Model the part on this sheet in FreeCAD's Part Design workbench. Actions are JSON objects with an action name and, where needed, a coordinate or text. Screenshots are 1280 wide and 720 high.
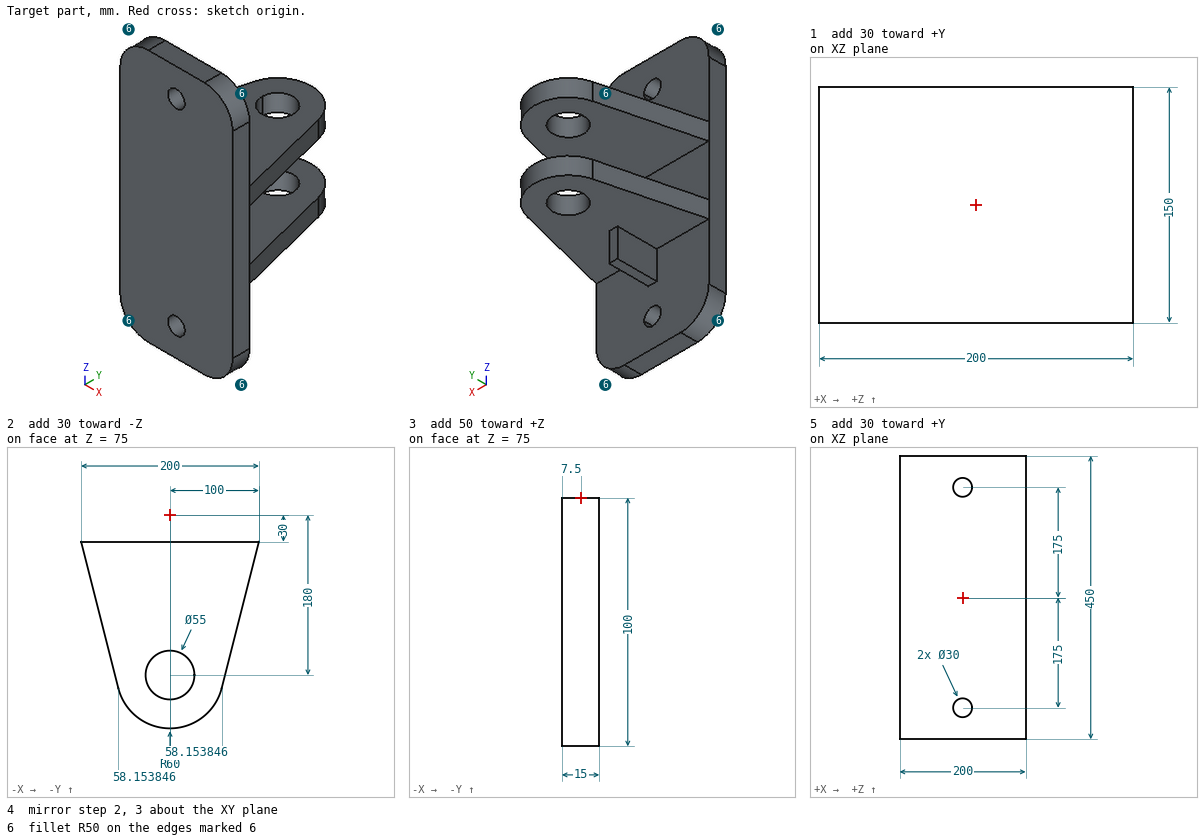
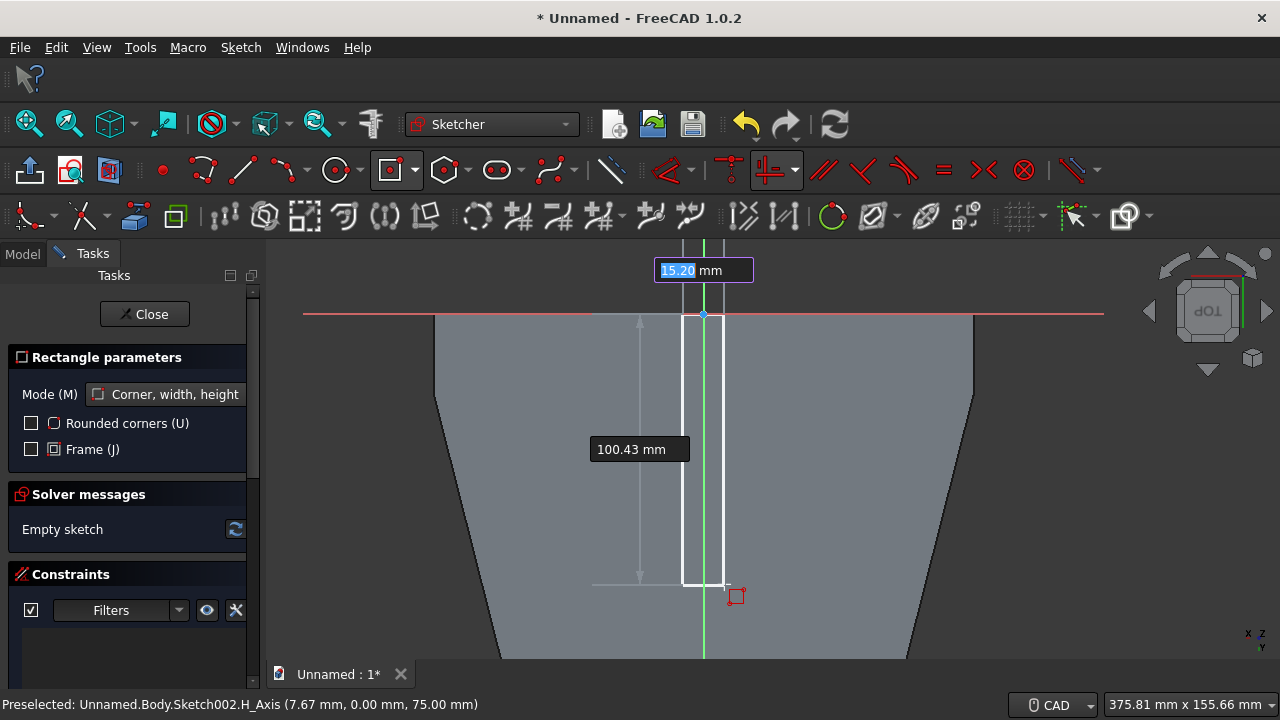
{"action": "type", "text": "15"}
{"action": "key", "text": "Tab"}
{"action": "type", "text": "100"}
{"action": "key", "text": "Return"}
{"action": "key", "text": "Escape"}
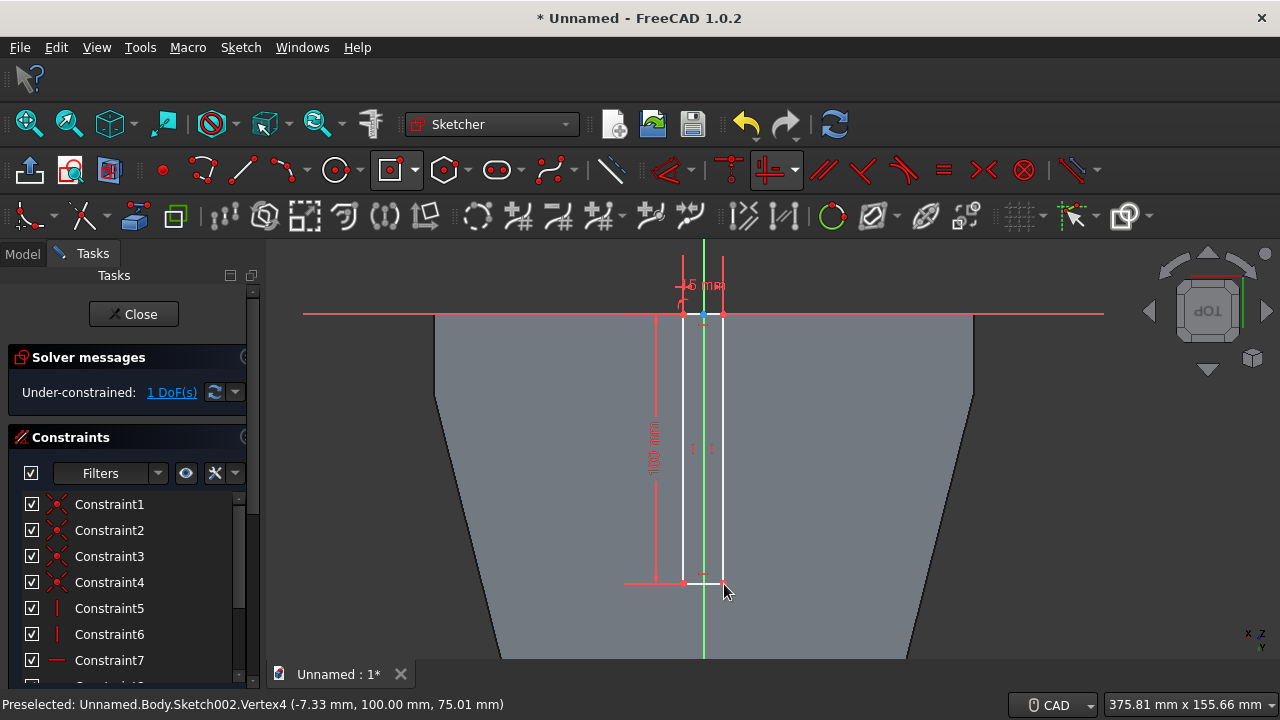
{"action": "key", "text": "d"}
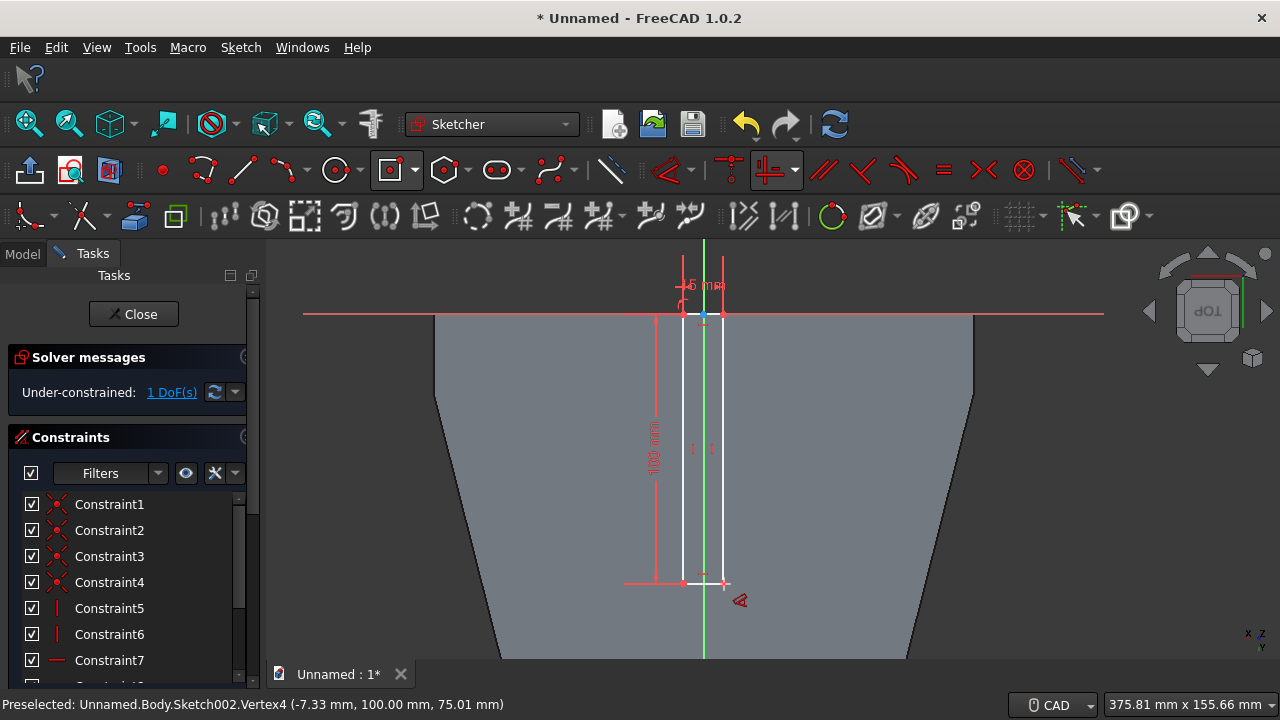
{"action": "scroll", "coordinate": [683, 314], "scroll_direction": "up", "scroll_amount": 4}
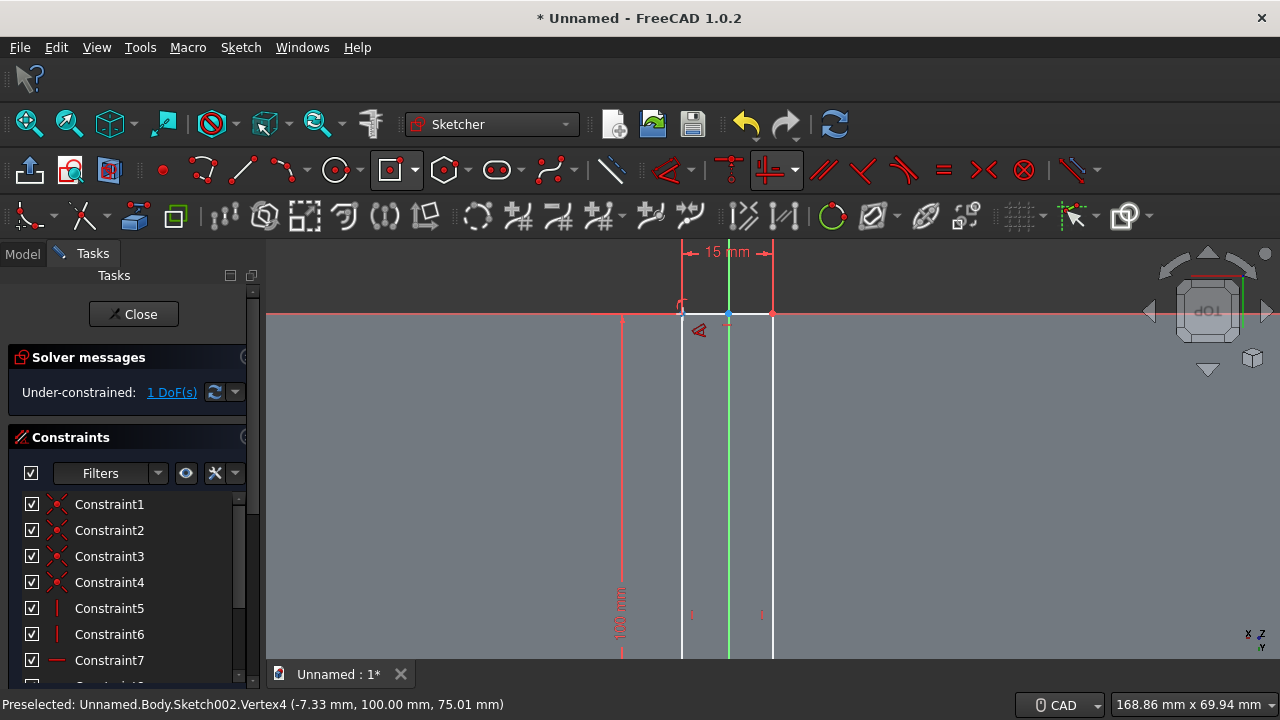
{"action": "left_click", "coordinate": [682, 314]}
{"action": "left_click", "coordinate": [706, 280]}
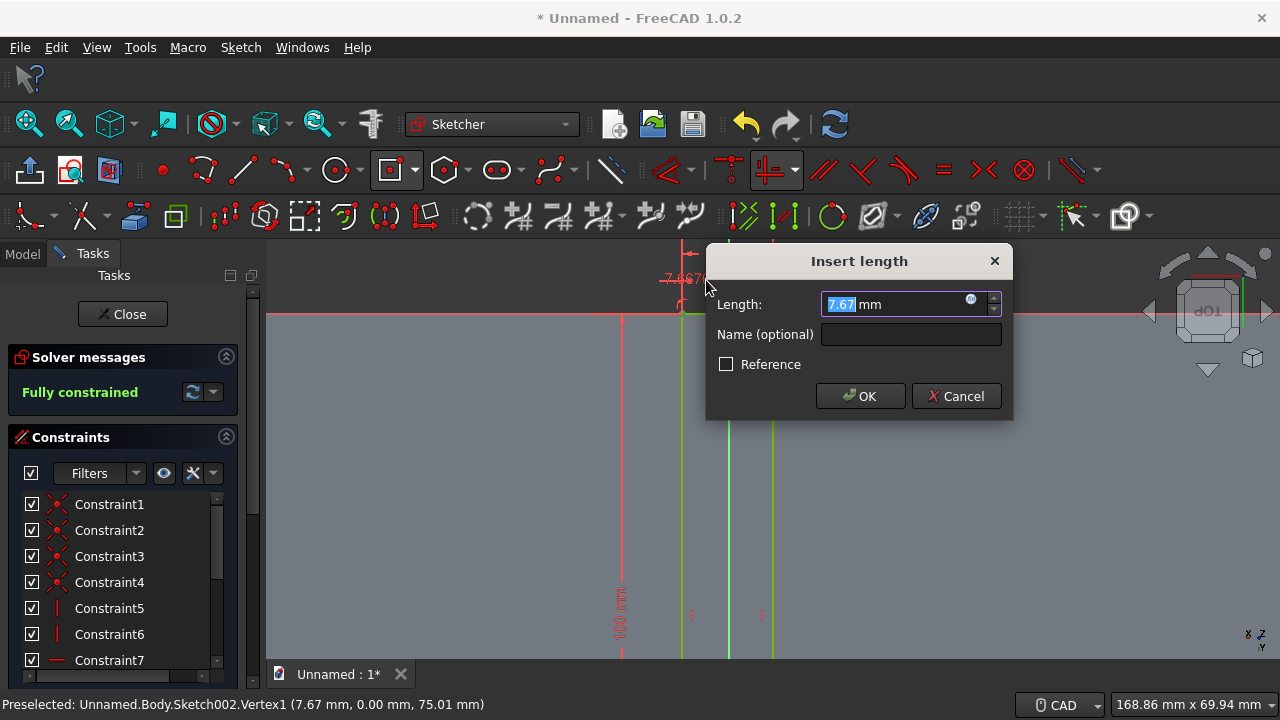
{"action": "type", "text": "7.5"}
{"action": "key", "text": "Return"}
{"action": "key", "text": "Escape"}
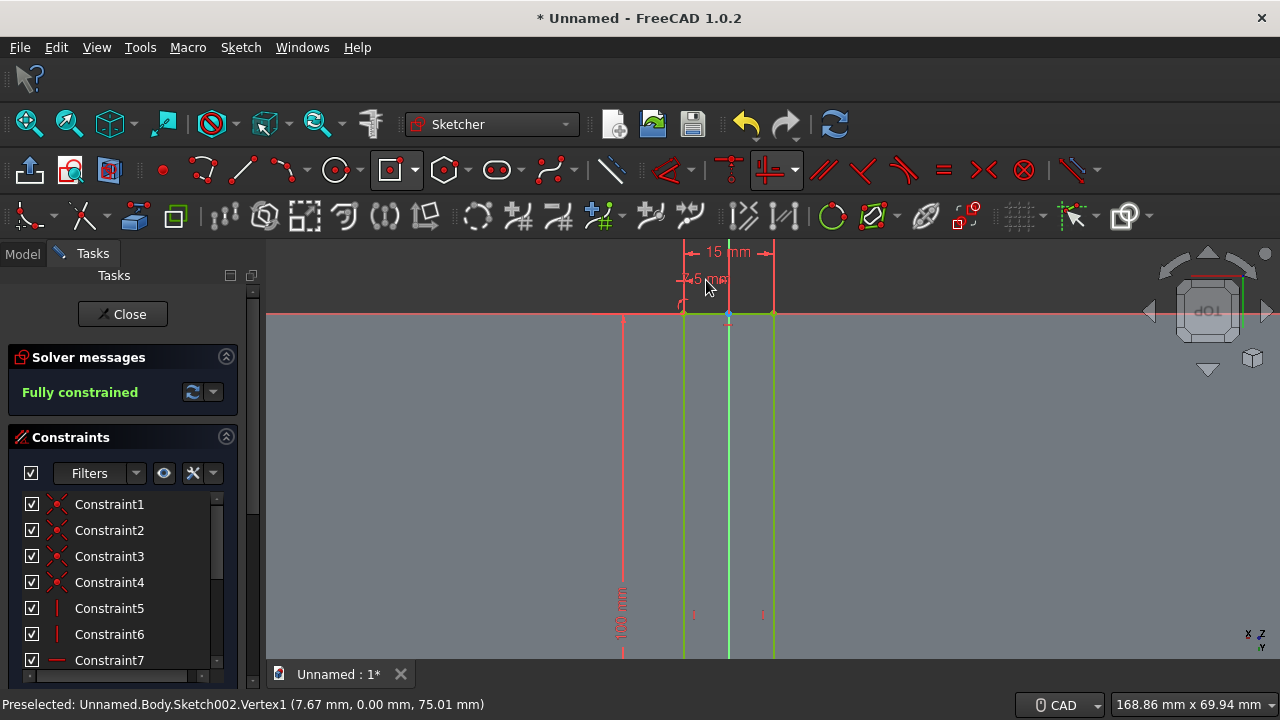
{"action": "left_click", "coordinate": [123, 314]}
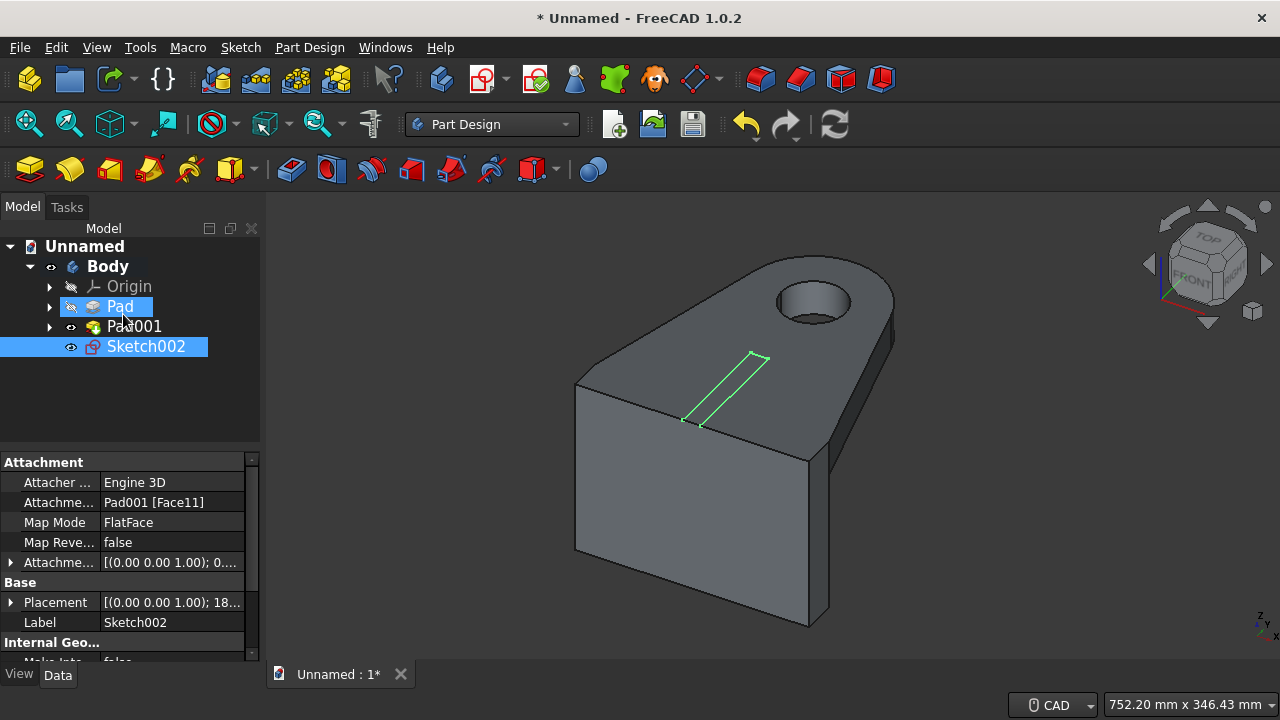
{"action": "left_click", "coordinate": [30, 170]}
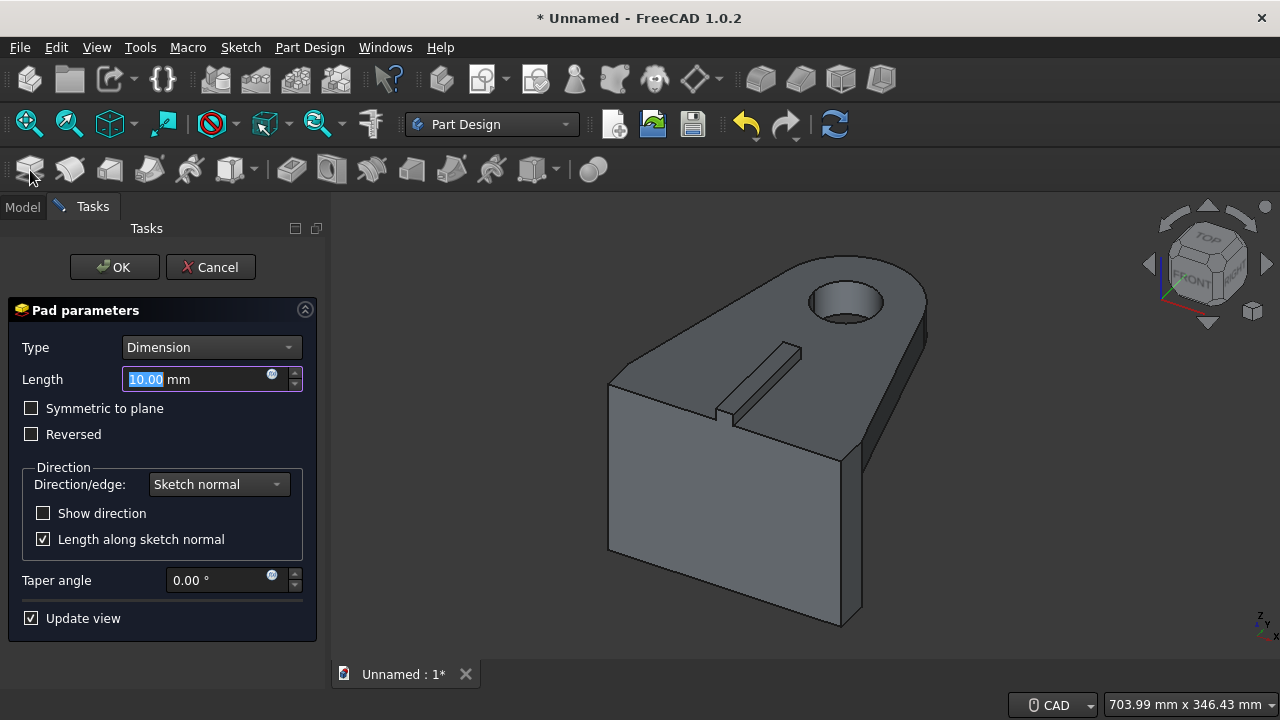
{"action": "type", "text": "50"}
{"action": "key", "text": "Tab"}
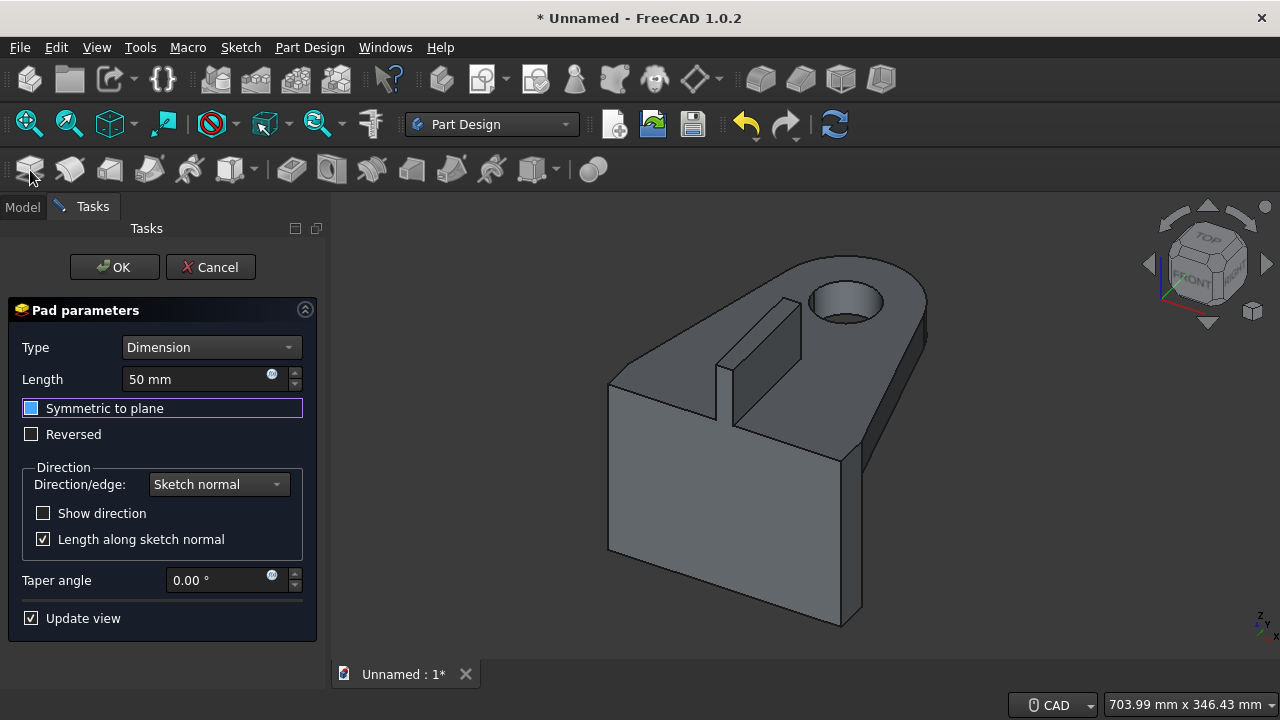
{"action": "left_click", "coordinate": [115, 267]}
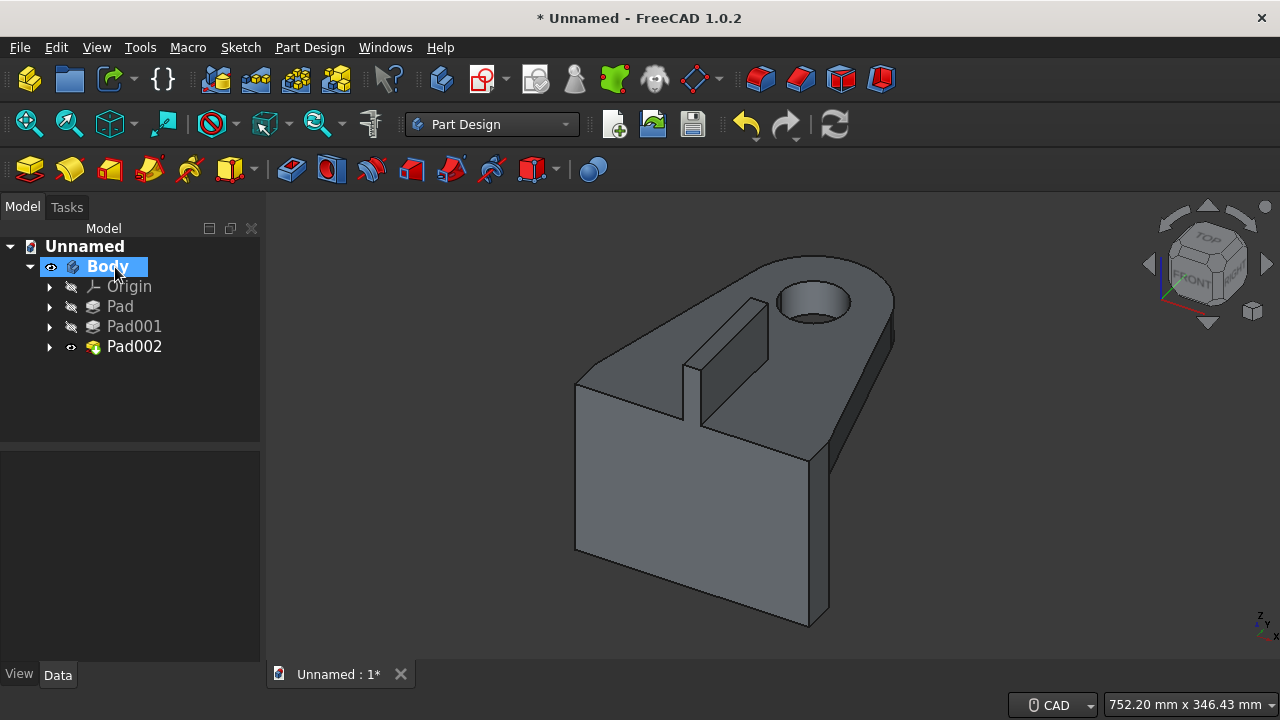
{"action": "key", "text": "v f"}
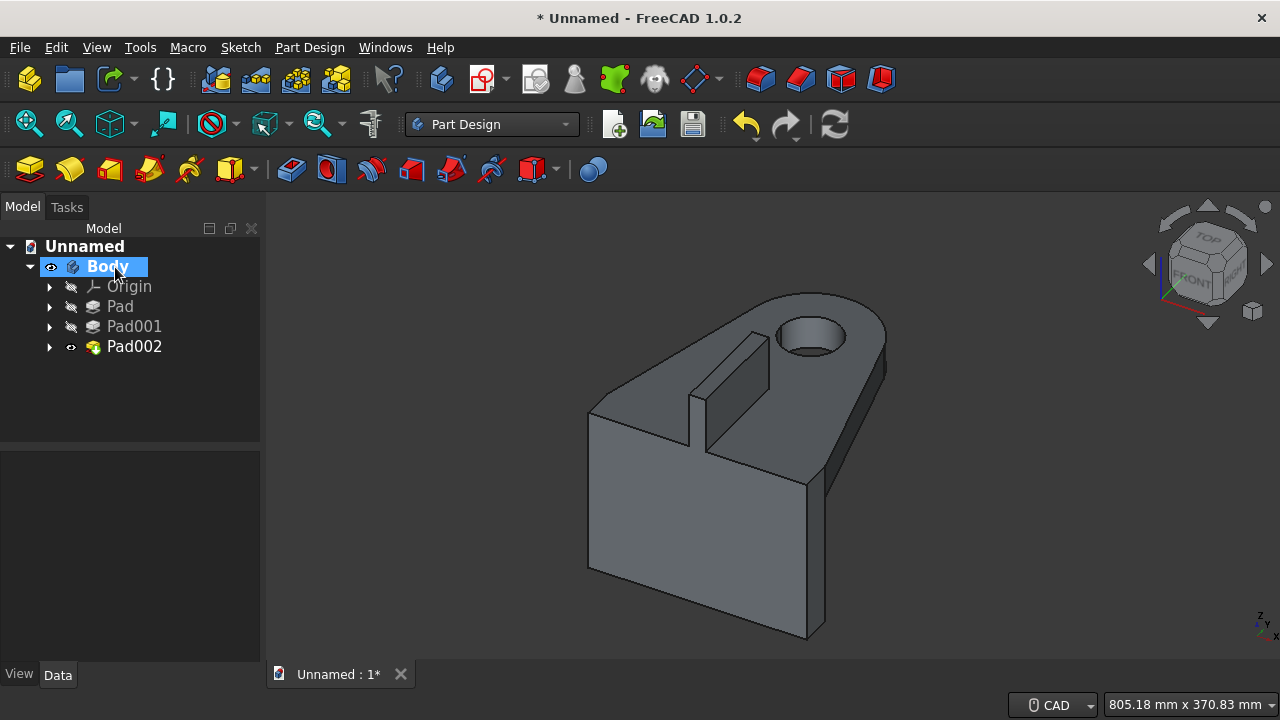
{"action": "left_click", "coordinate": [116, 327]}